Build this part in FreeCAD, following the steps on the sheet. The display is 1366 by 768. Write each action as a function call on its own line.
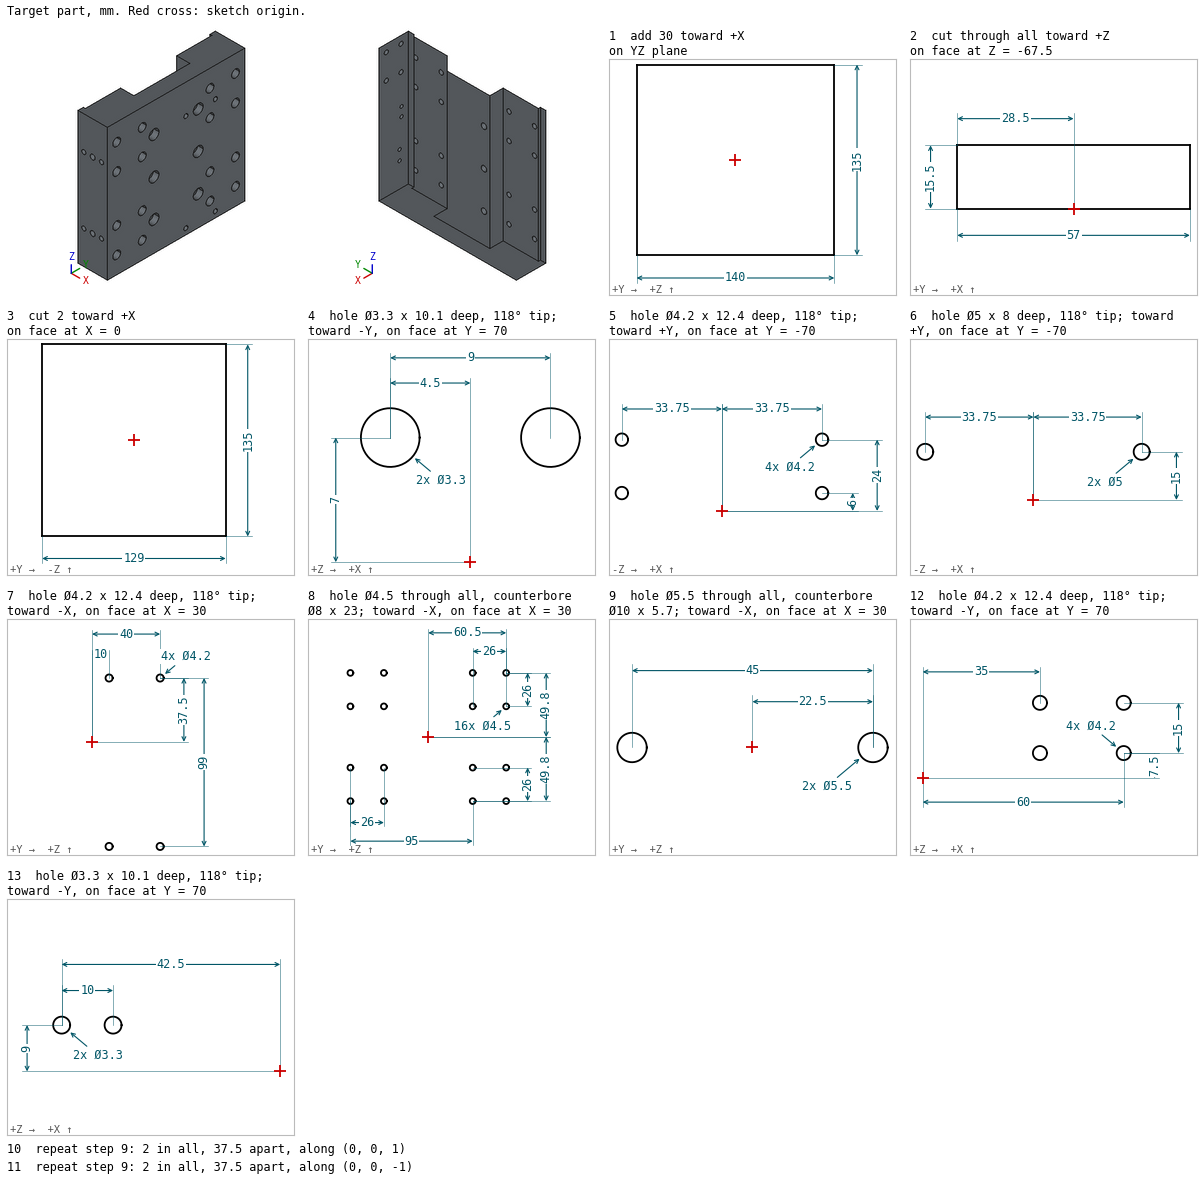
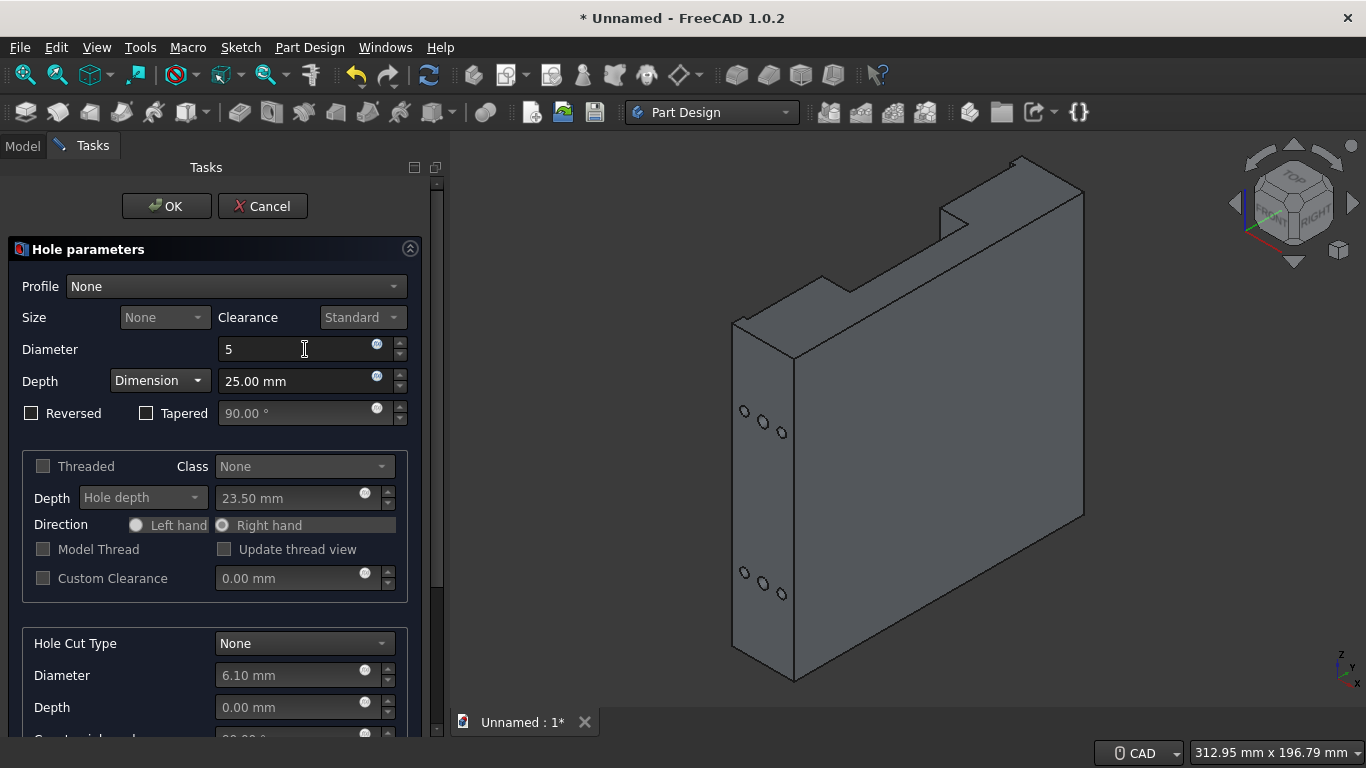
triple_click(305, 381)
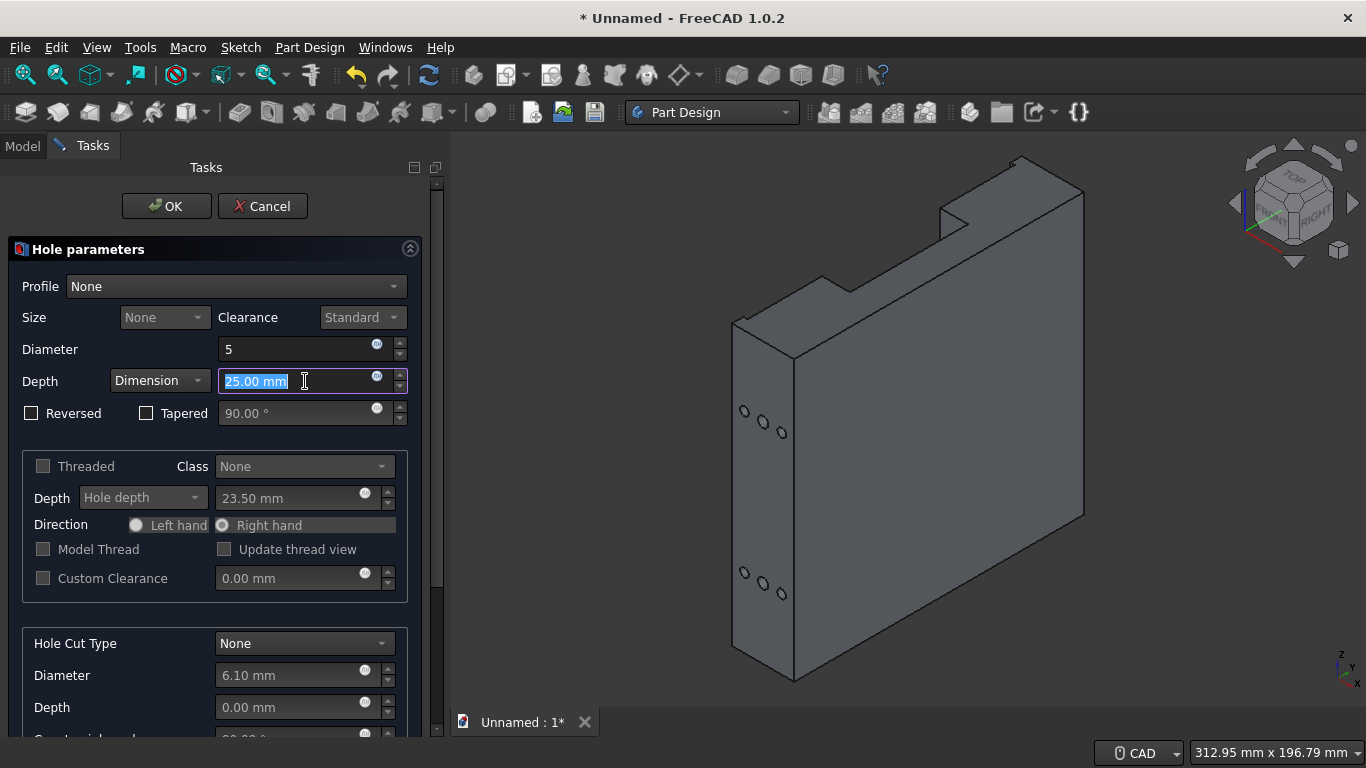
text(8)
key(Tab)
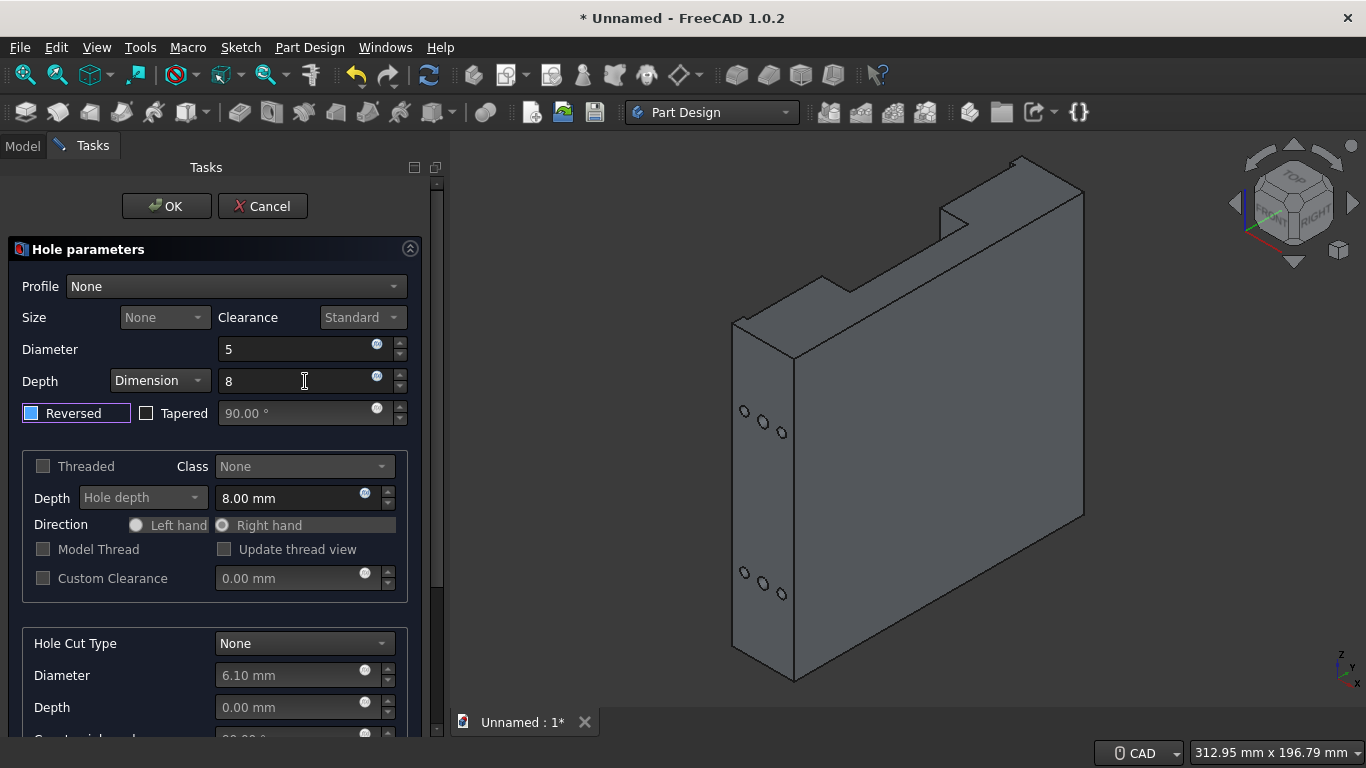
click(167, 206)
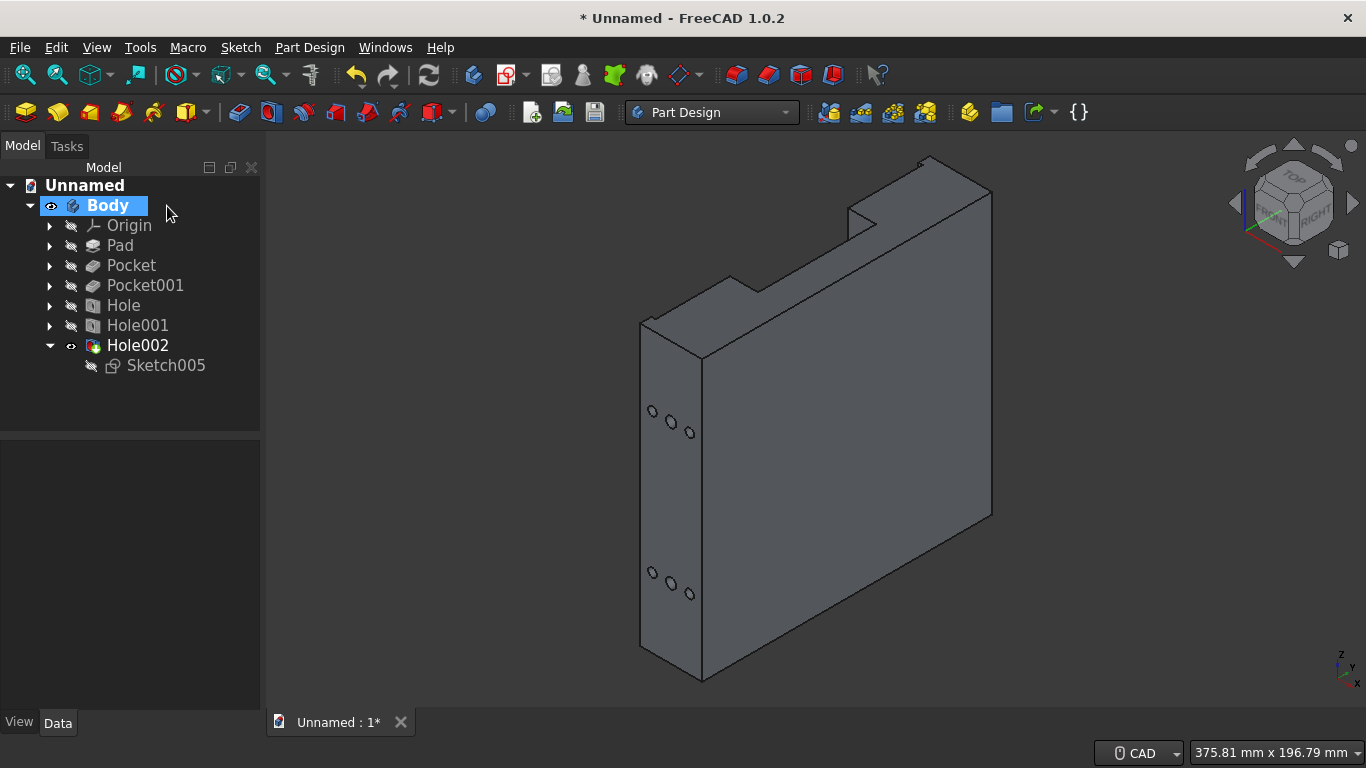
click(847, 436)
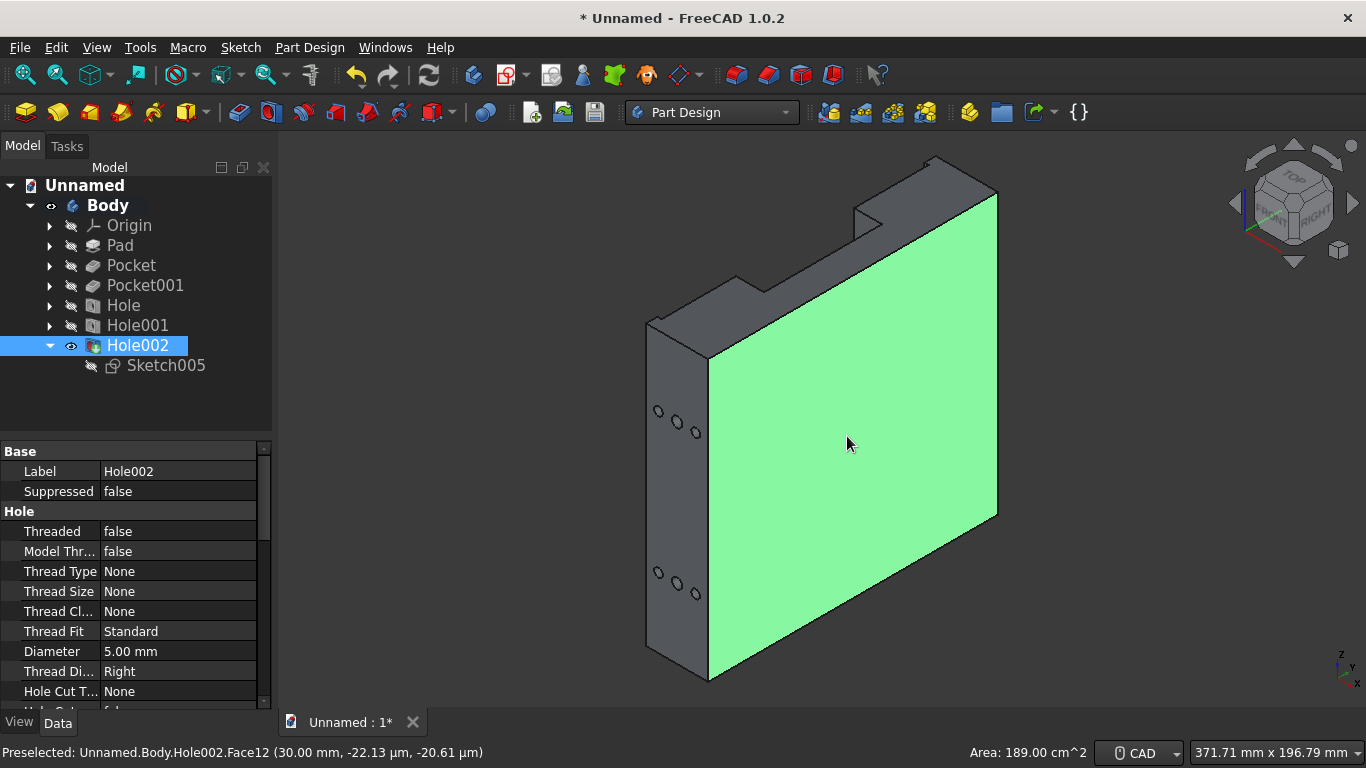
click(506, 76)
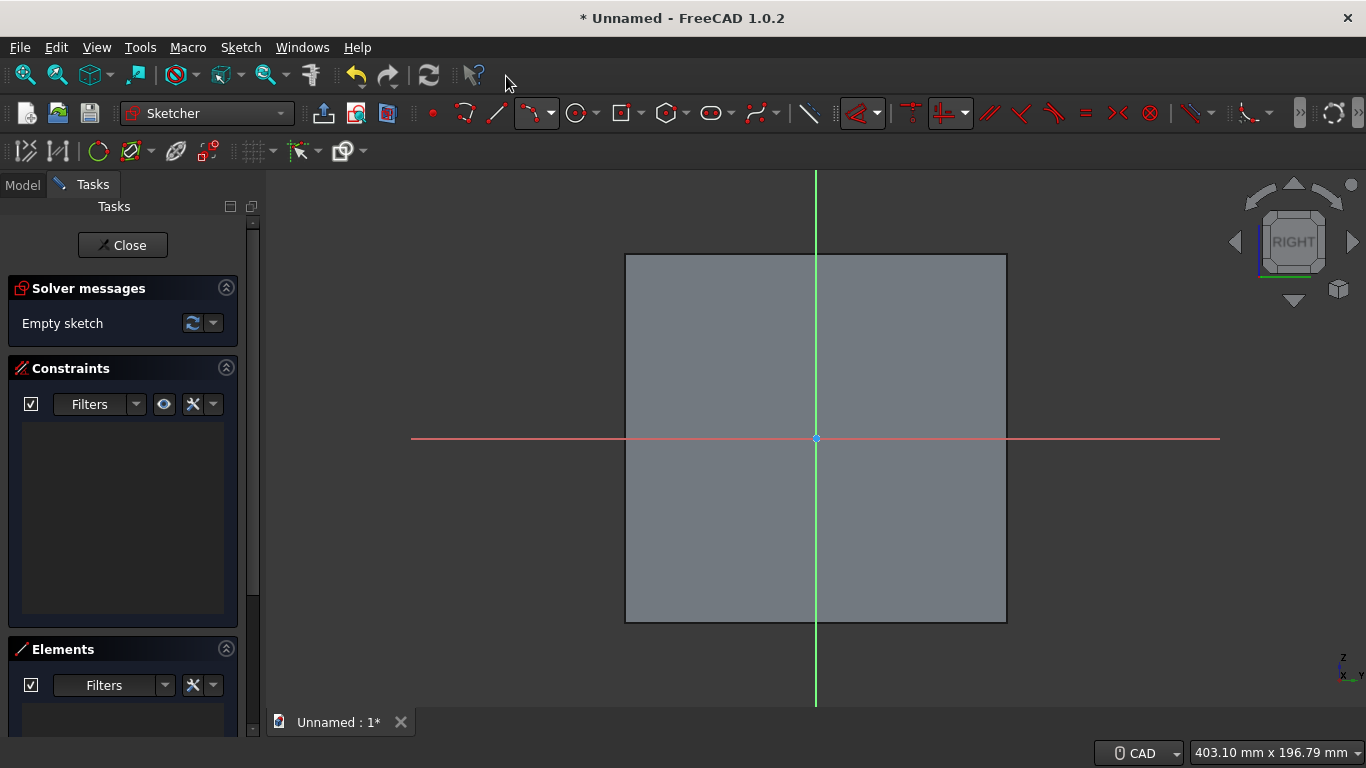
click(576, 114)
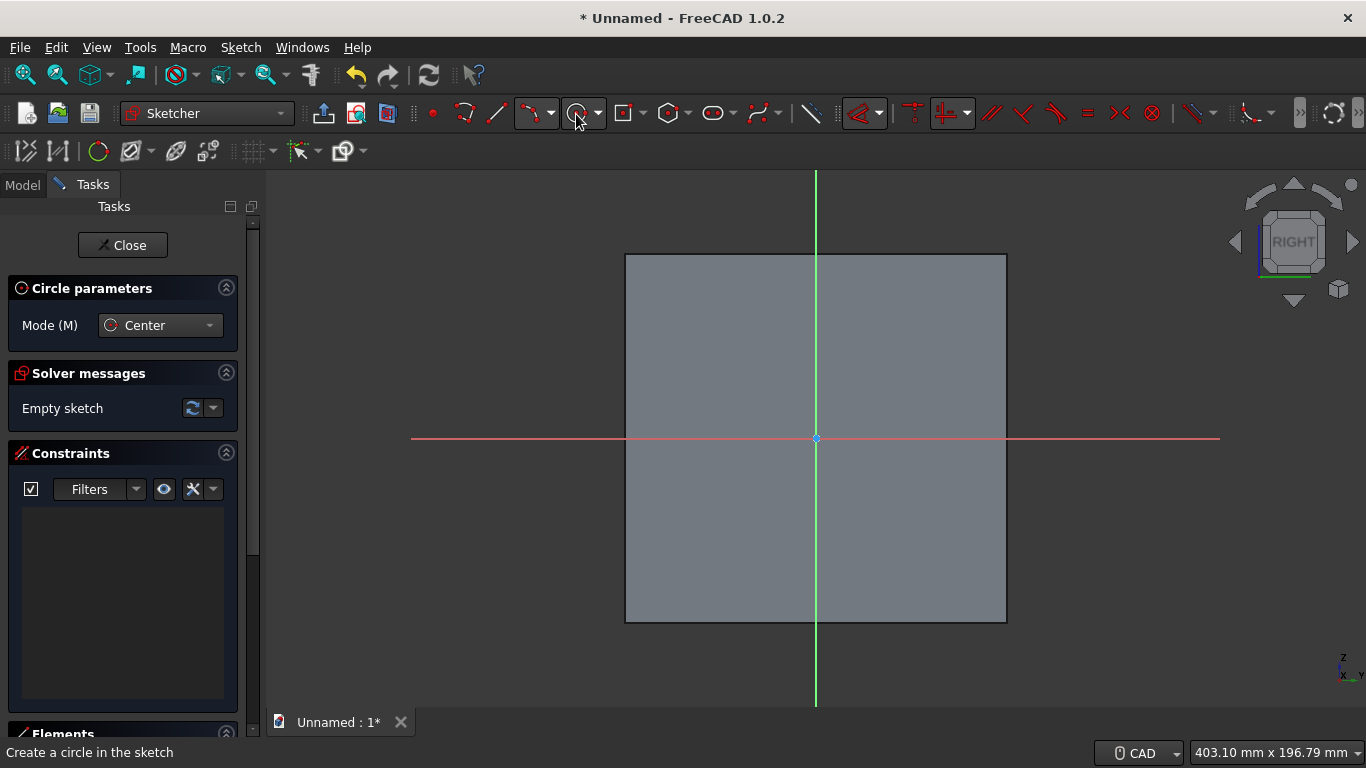
scroll(925, 336, up, 7)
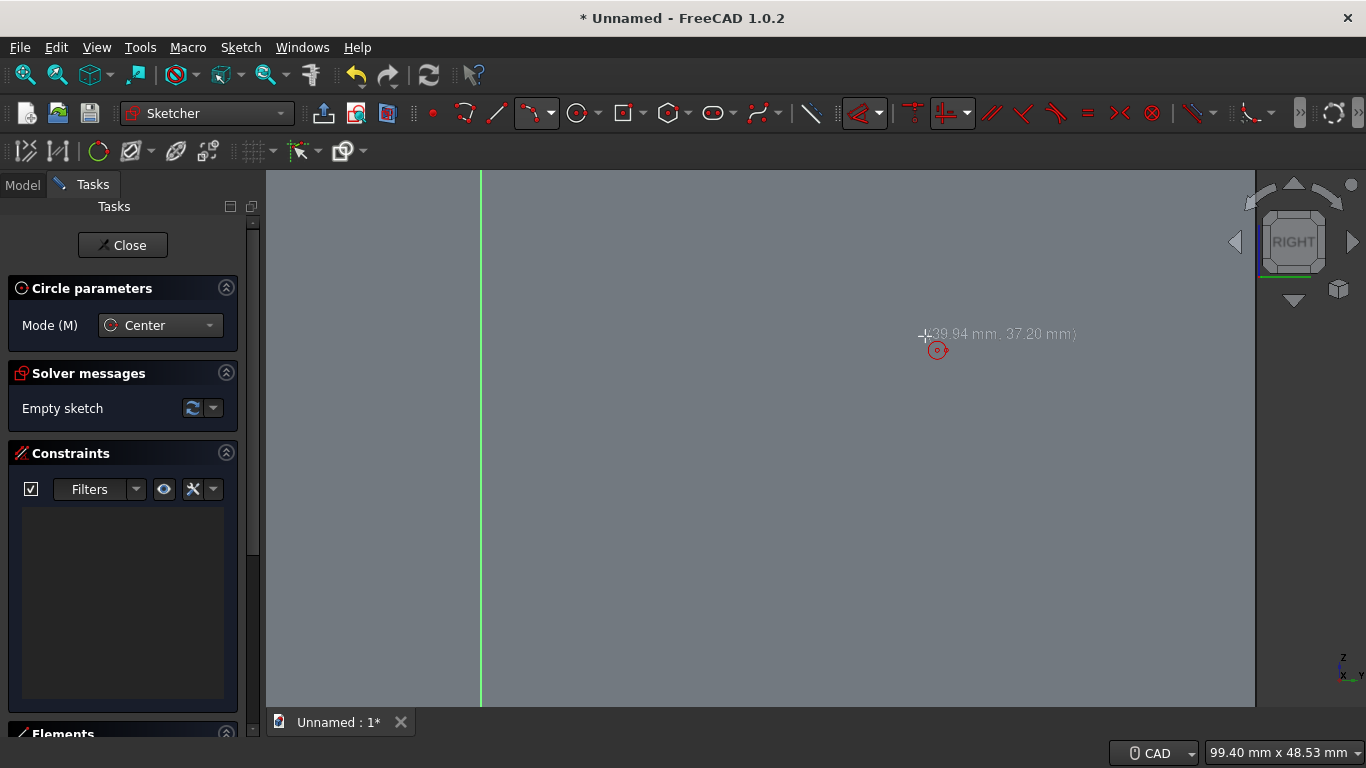
scroll(762, 247, down, 6)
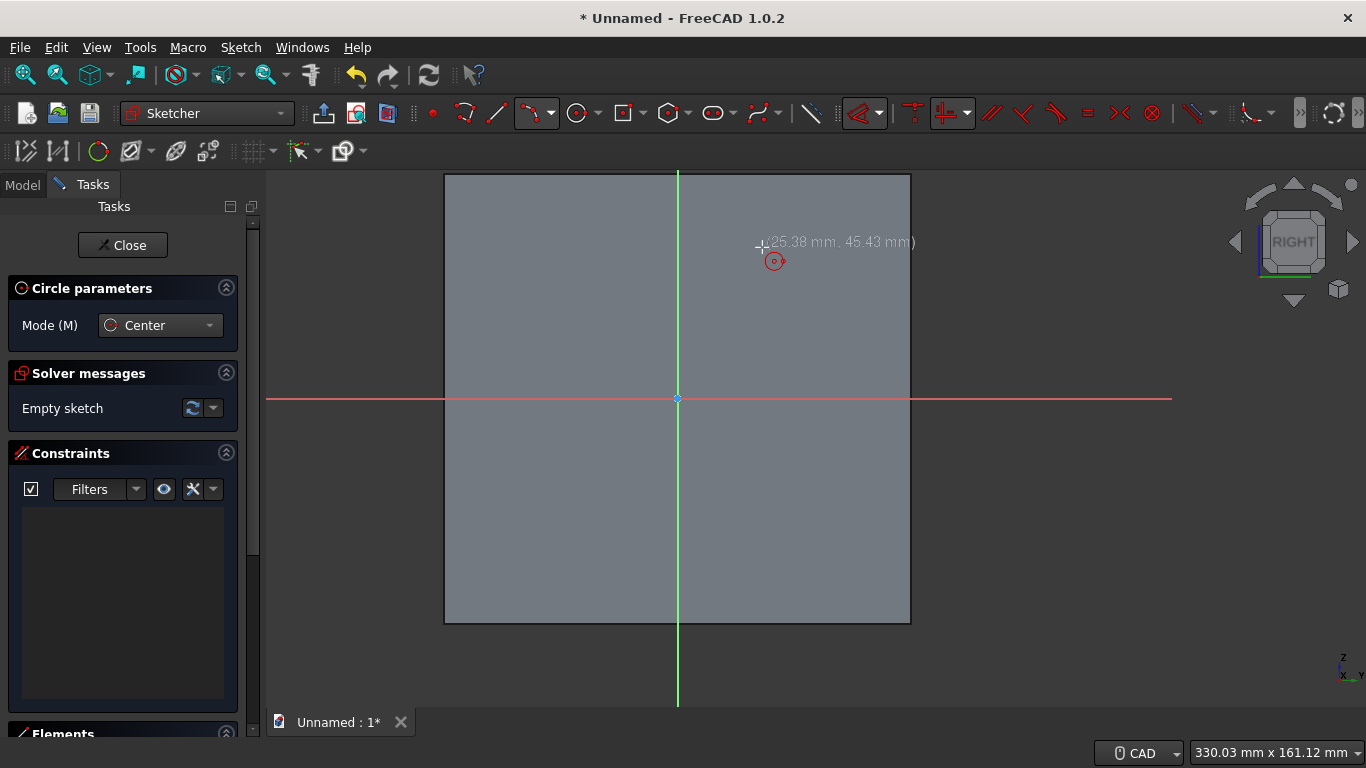
click(811, 274)